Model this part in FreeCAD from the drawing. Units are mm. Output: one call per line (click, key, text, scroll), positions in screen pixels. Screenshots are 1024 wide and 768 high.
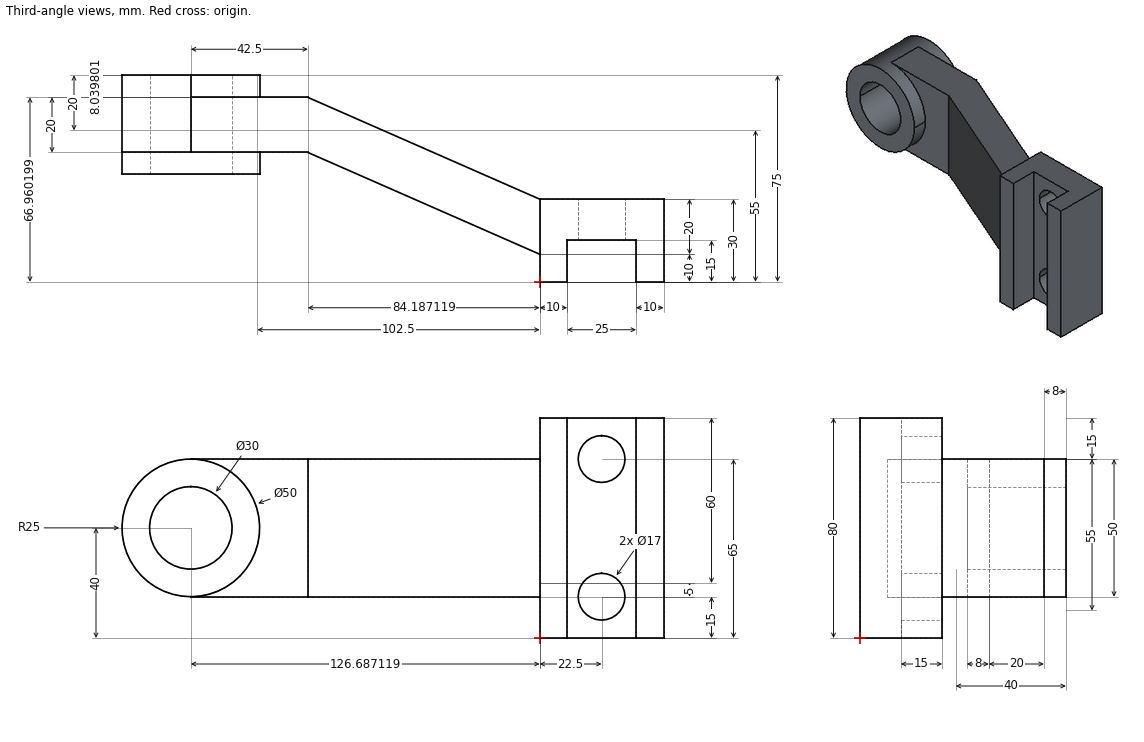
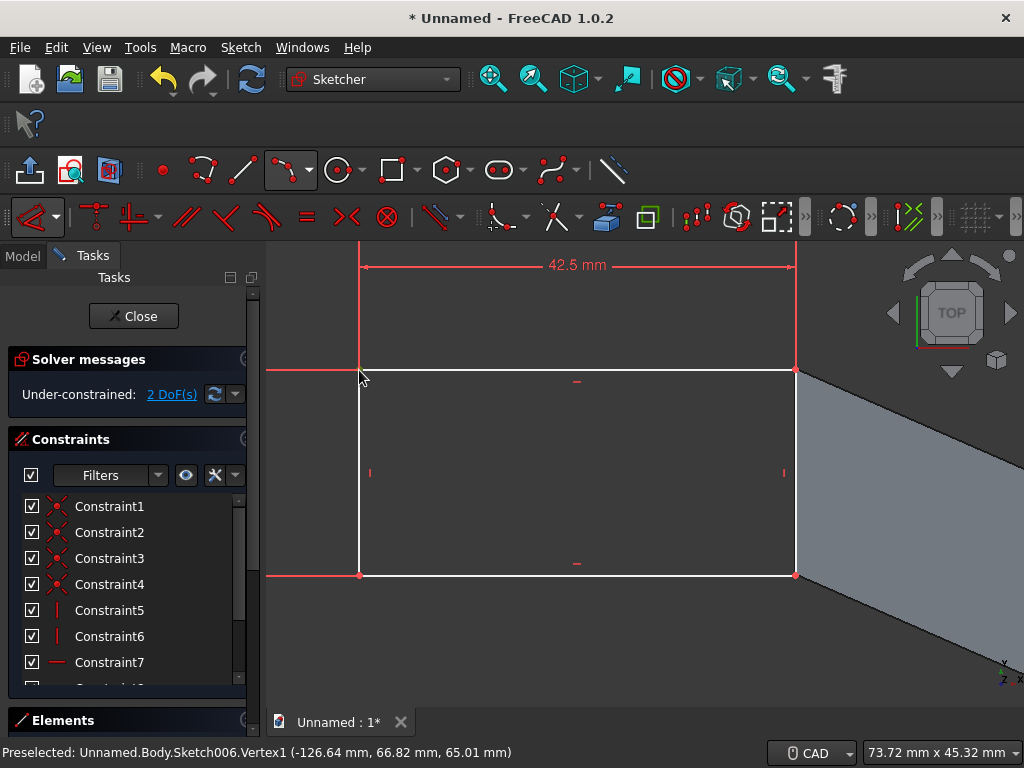
key(i)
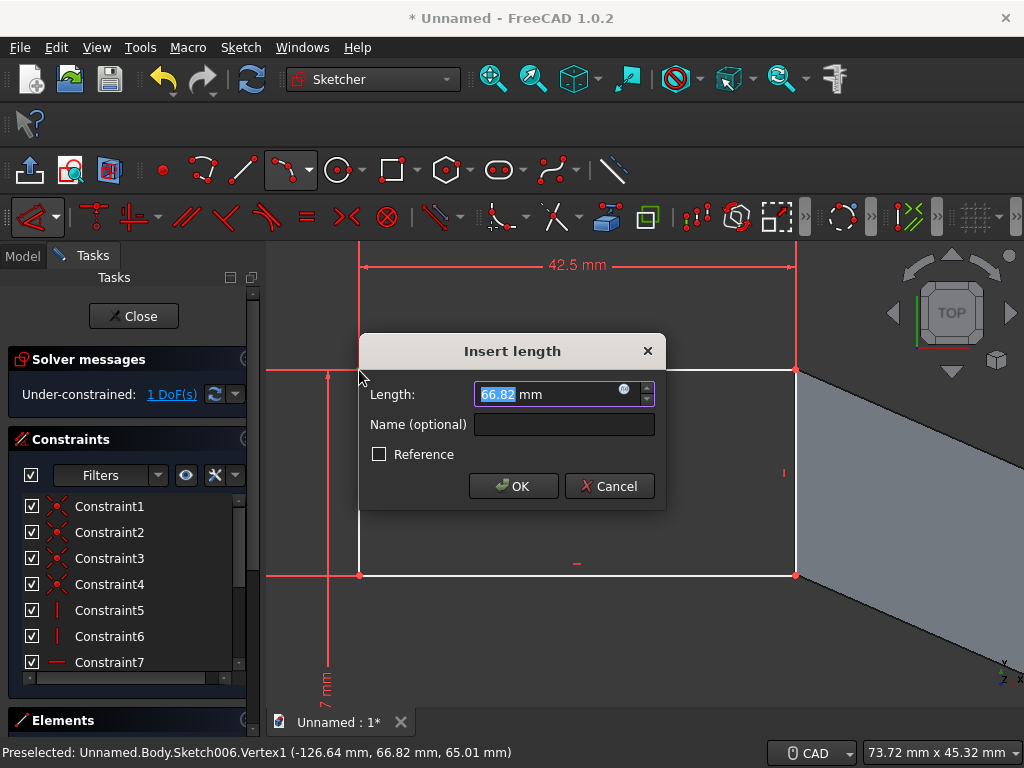
text(66.960199)
key(Return)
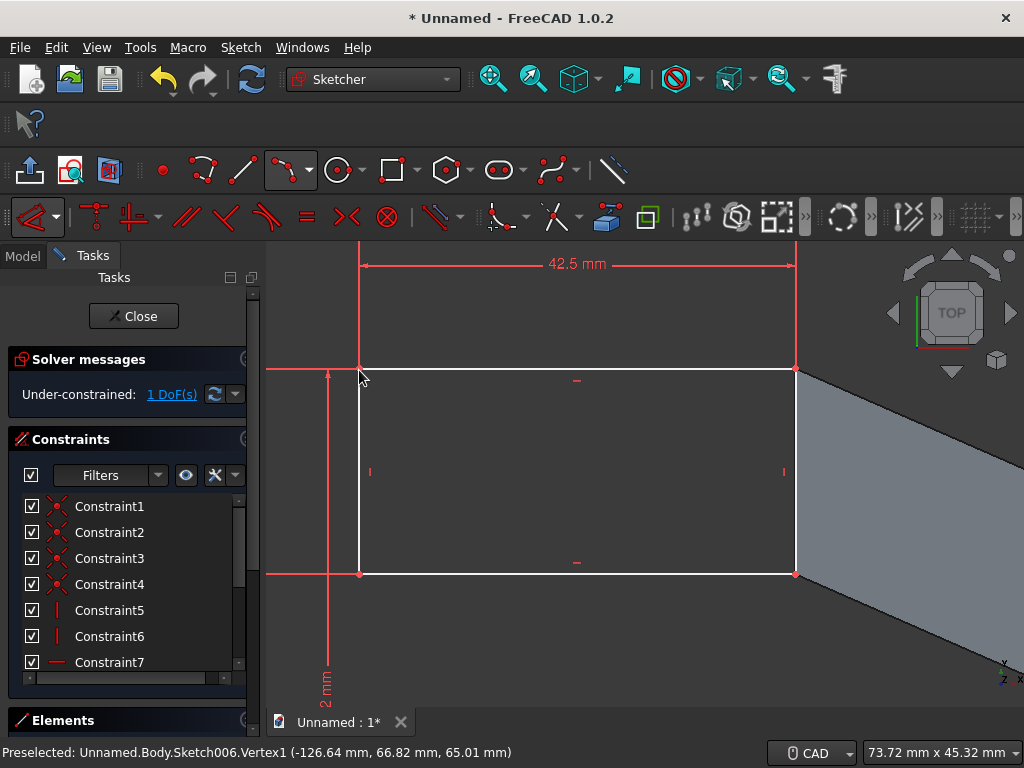
click(796, 574)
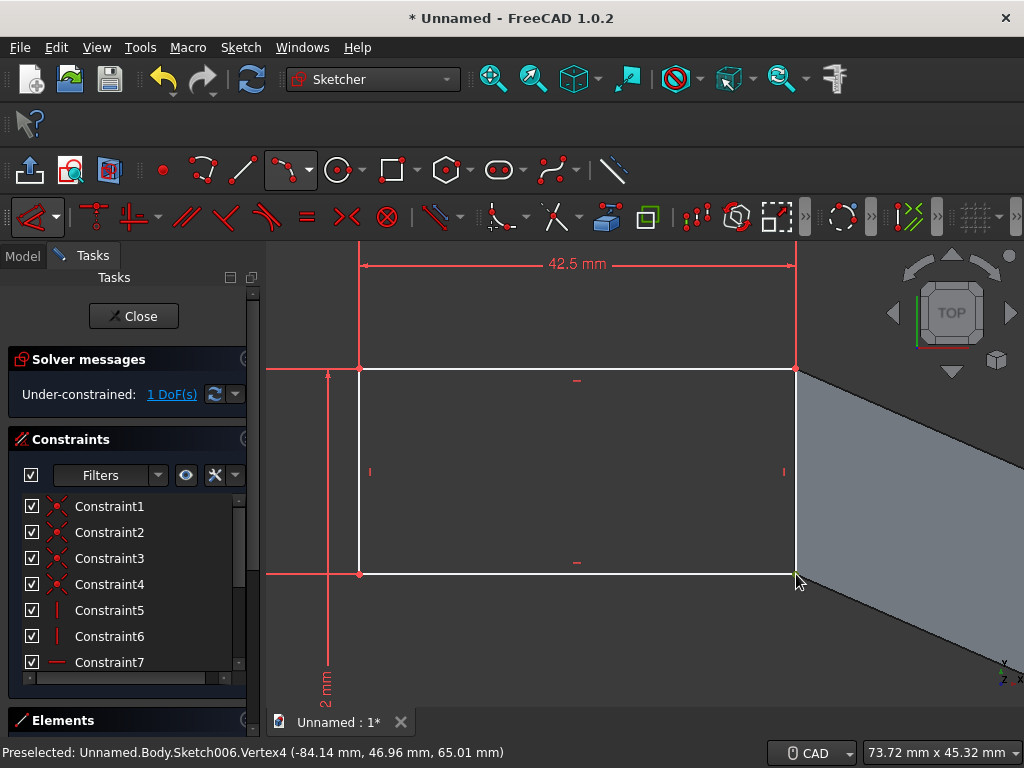
click(58, 218)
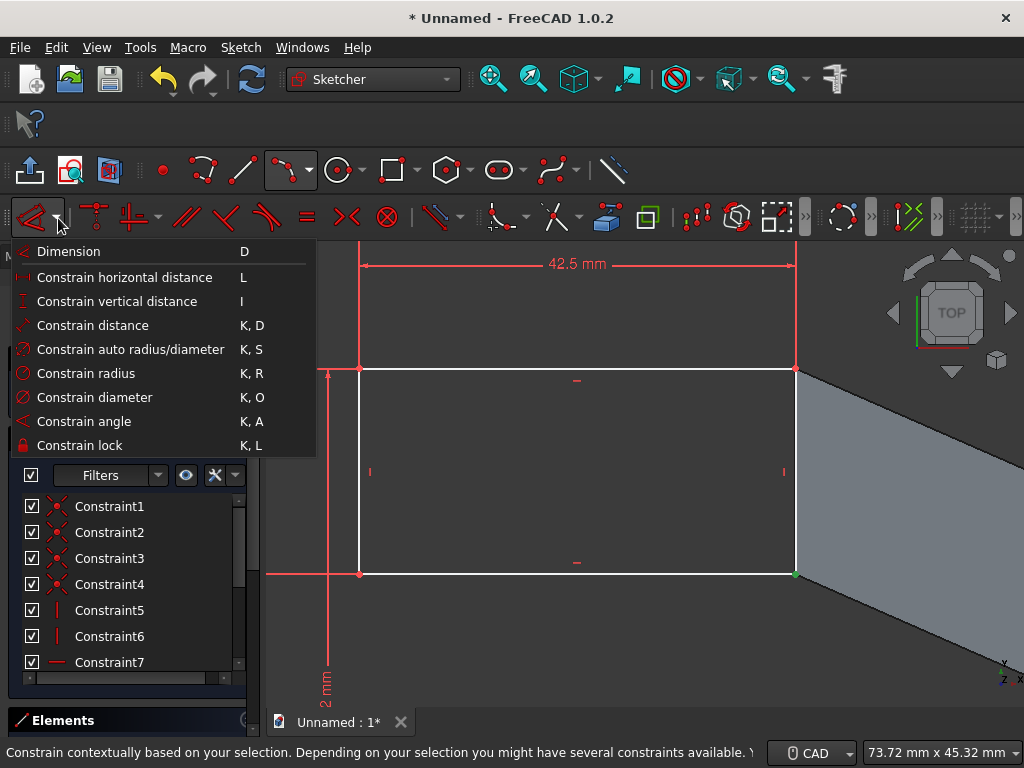
click(164, 277)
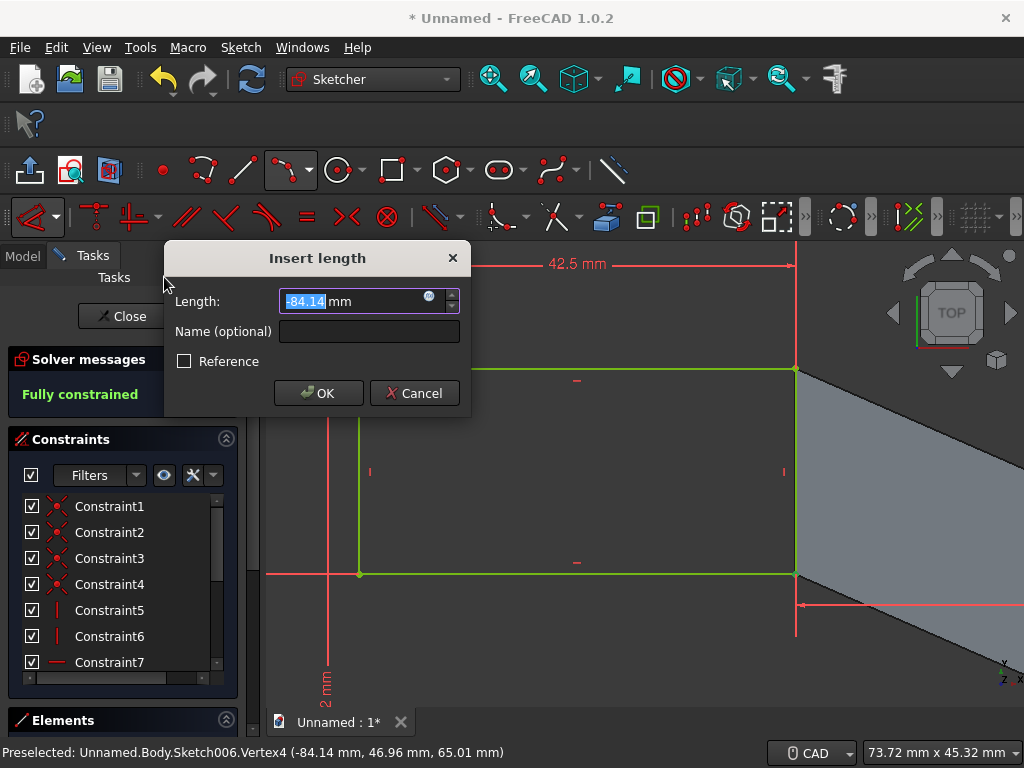
text(-84.187119)
key(Return)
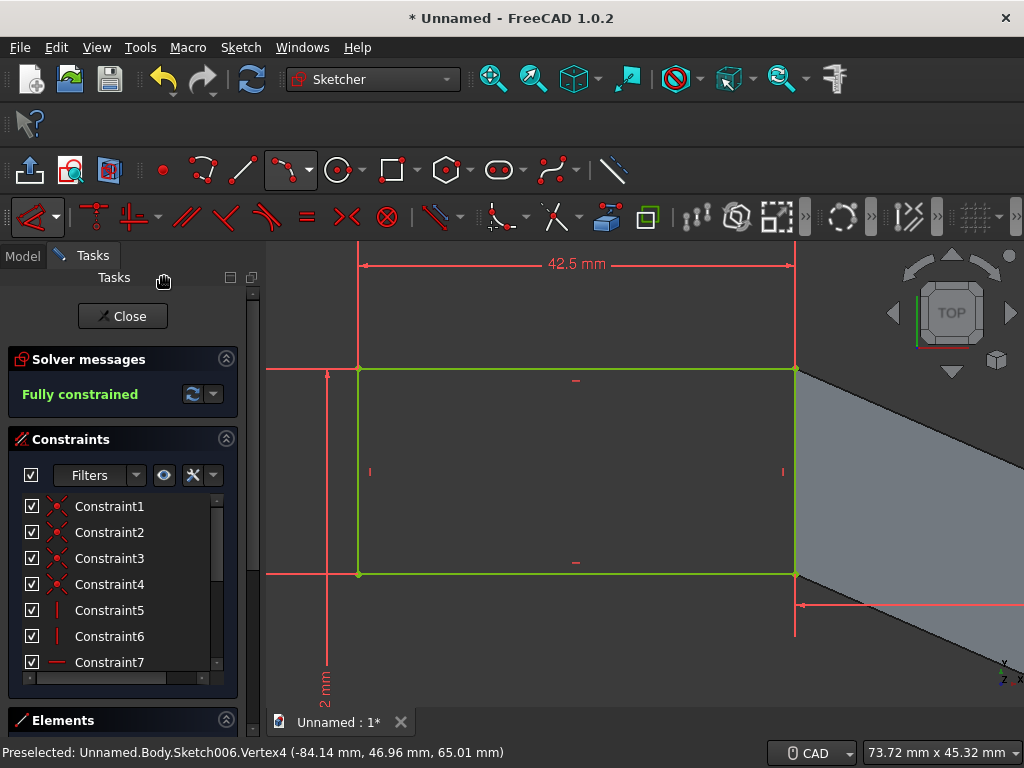
click(123, 316)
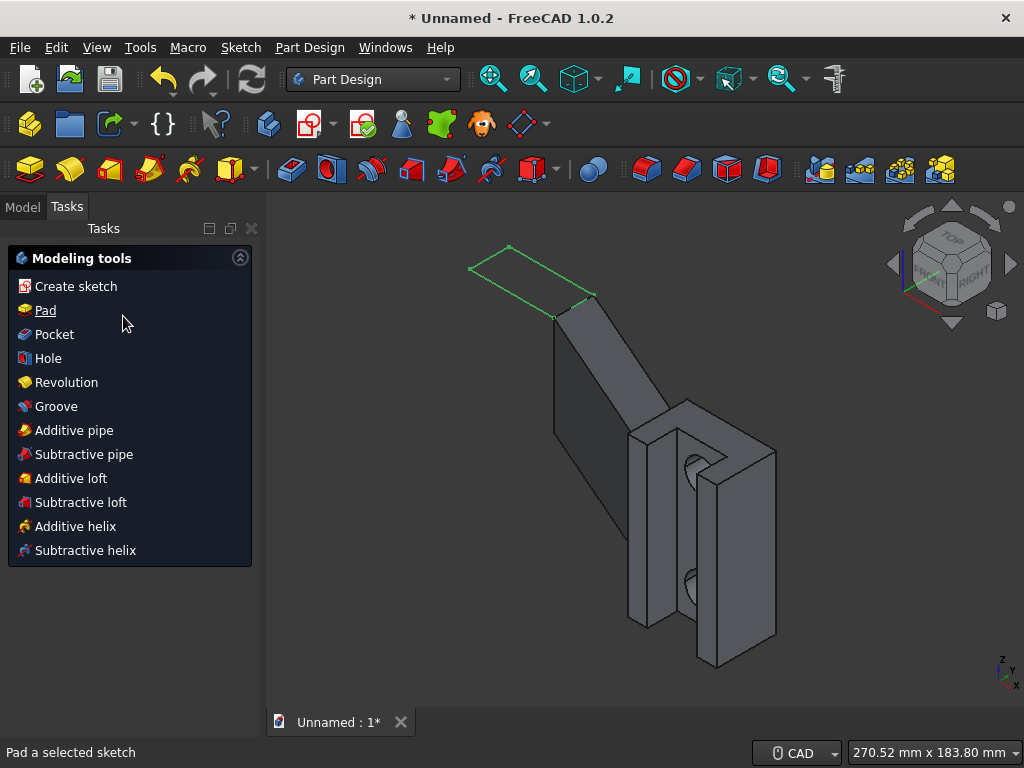
click(30, 170)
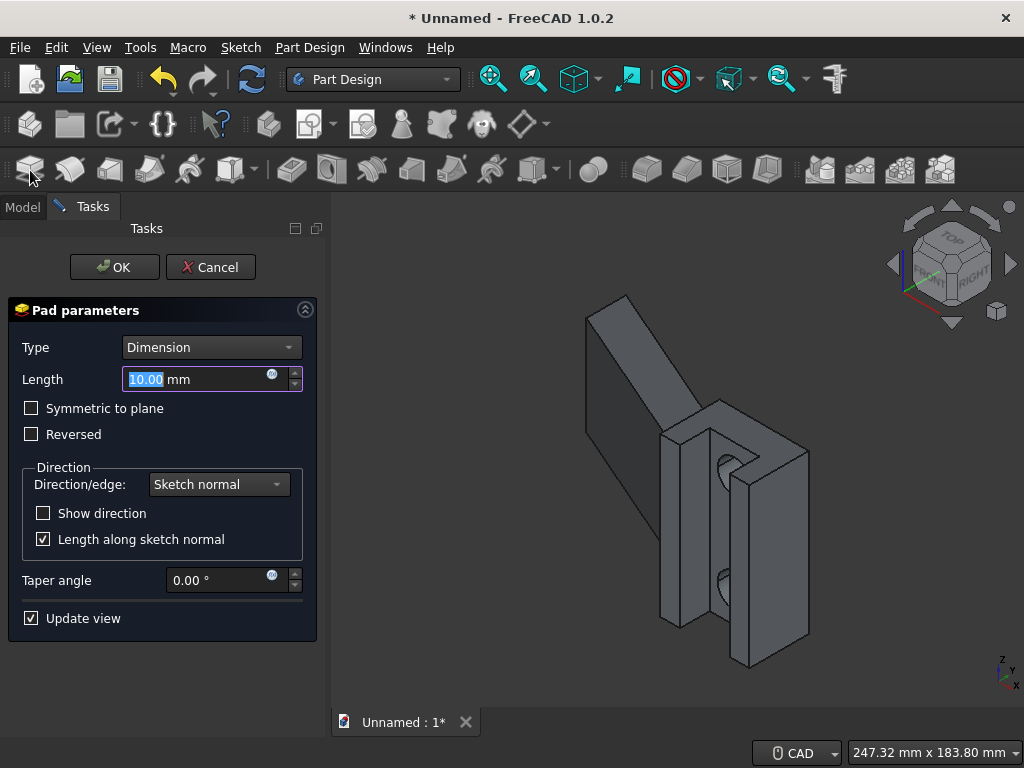
text(50)
key(Tab)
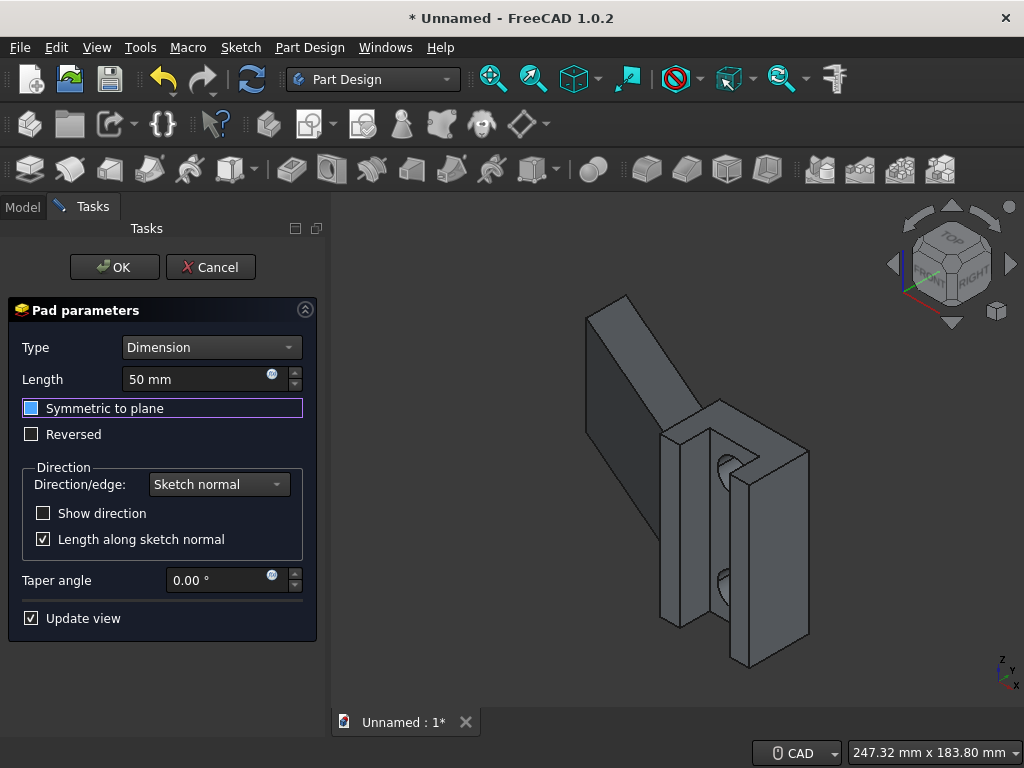
click(30, 434)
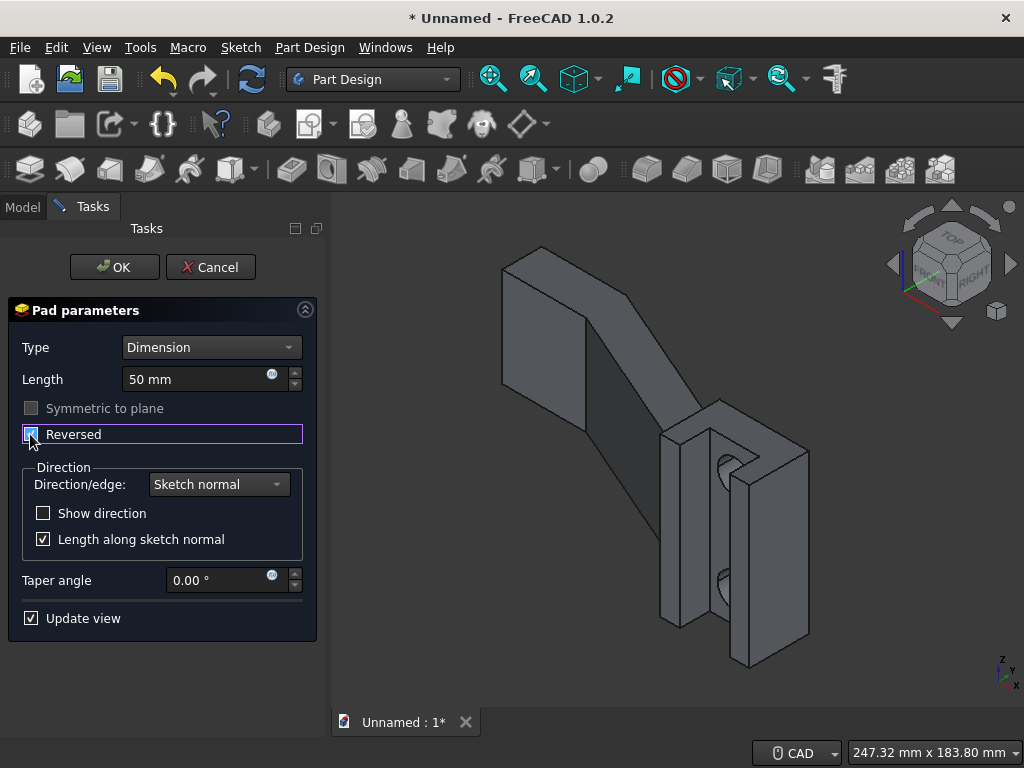
click(115, 267)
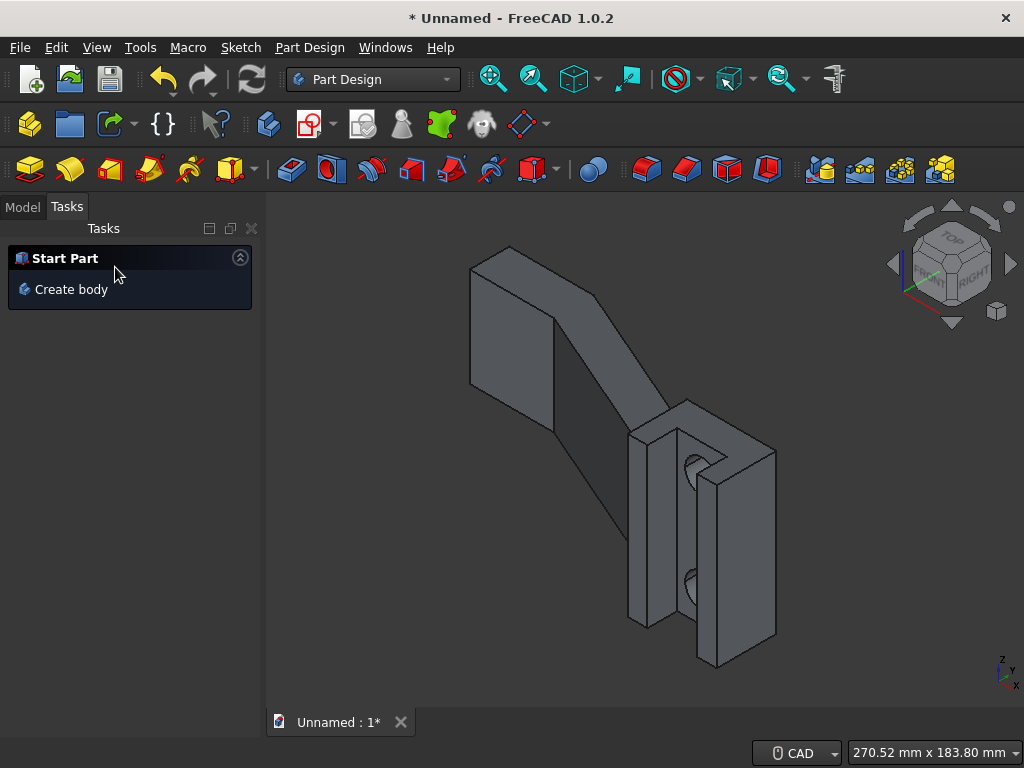
key(4)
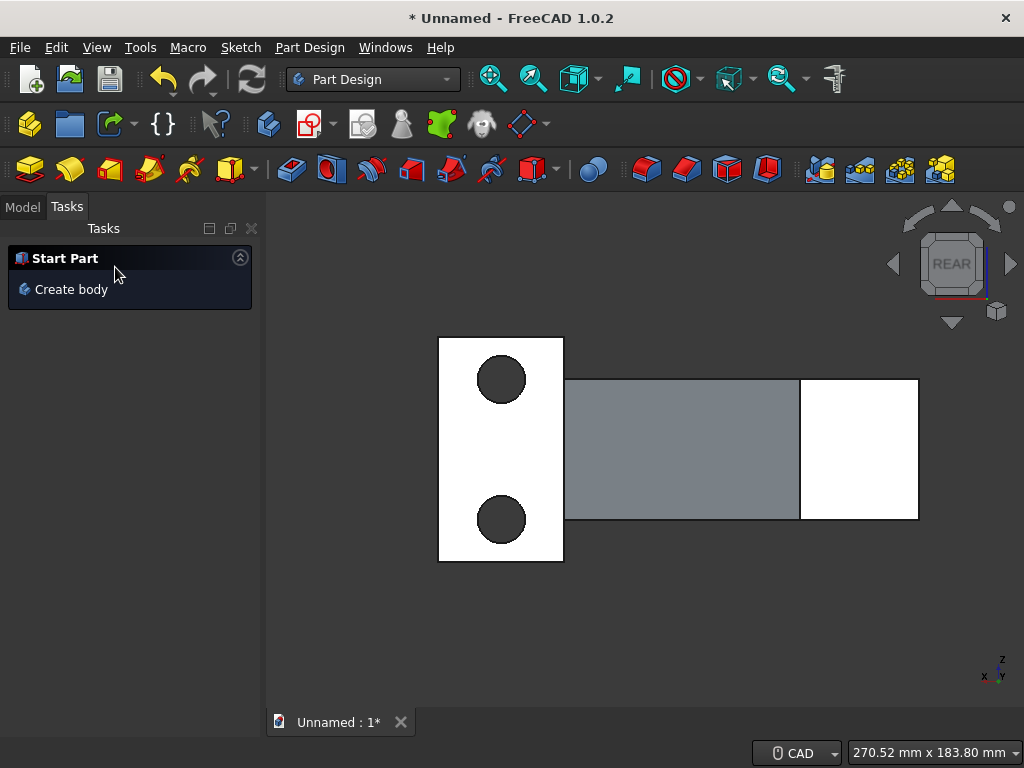
click(860, 449)